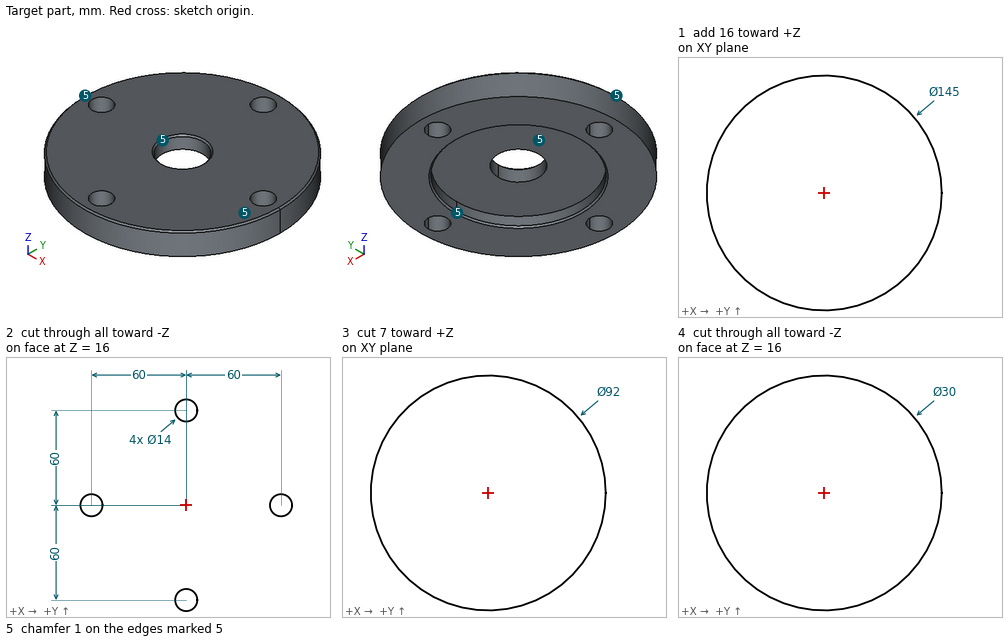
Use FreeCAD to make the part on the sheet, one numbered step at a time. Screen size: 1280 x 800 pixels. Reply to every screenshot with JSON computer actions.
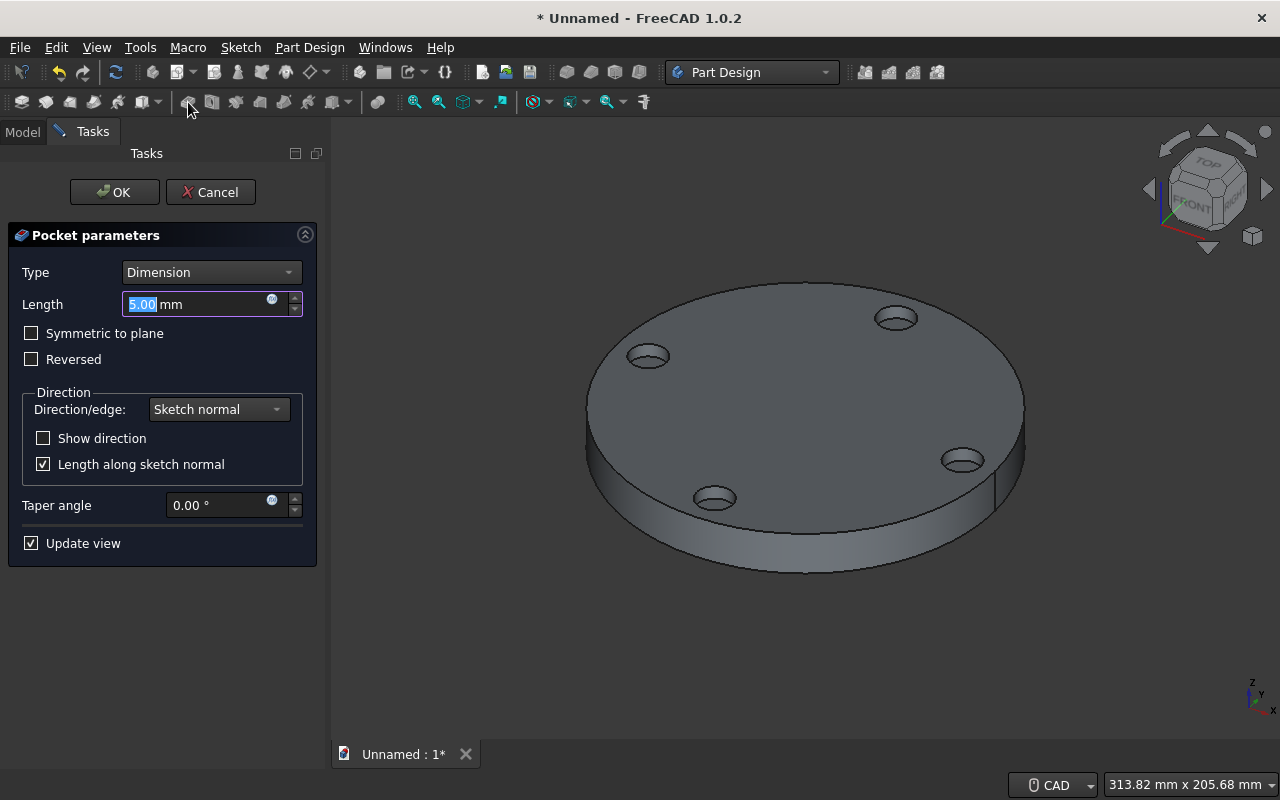
{"action": "left_click", "coordinate": [212, 272]}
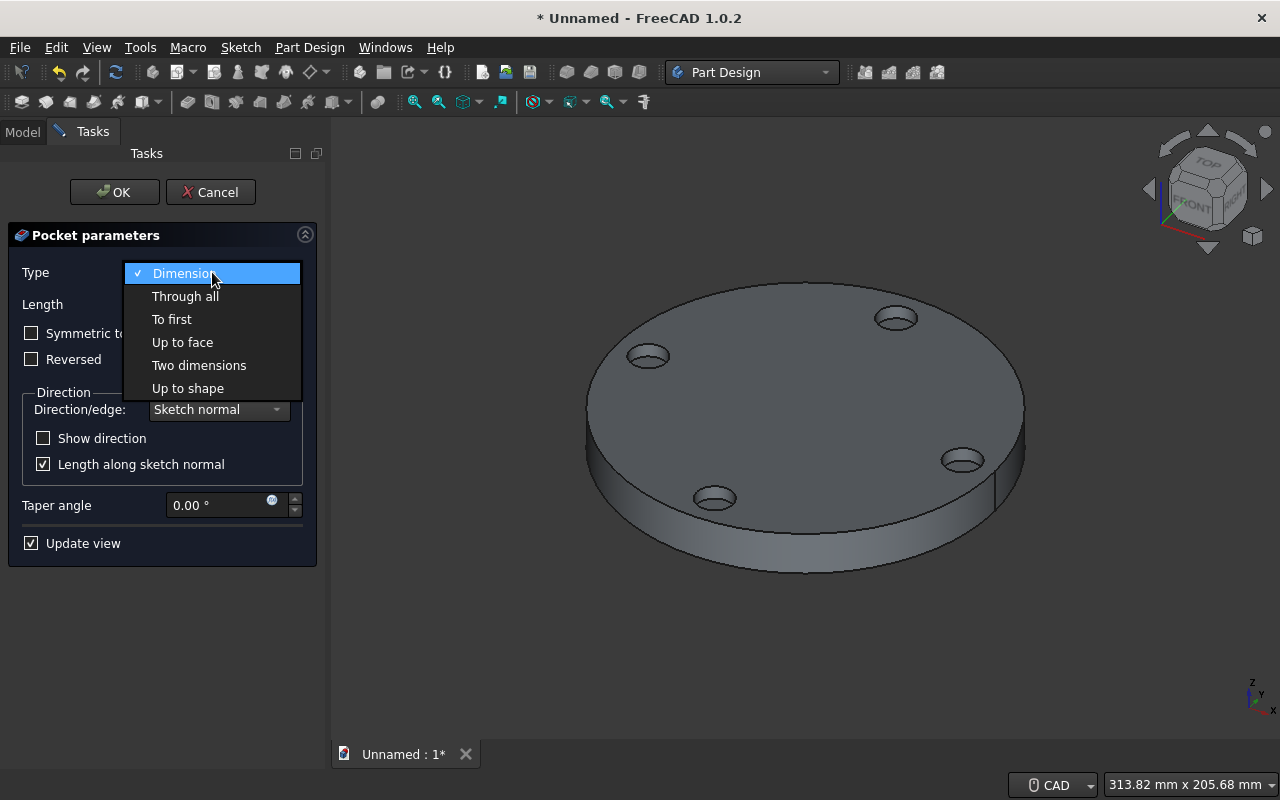
{"action": "left_click", "coordinate": [212, 296]}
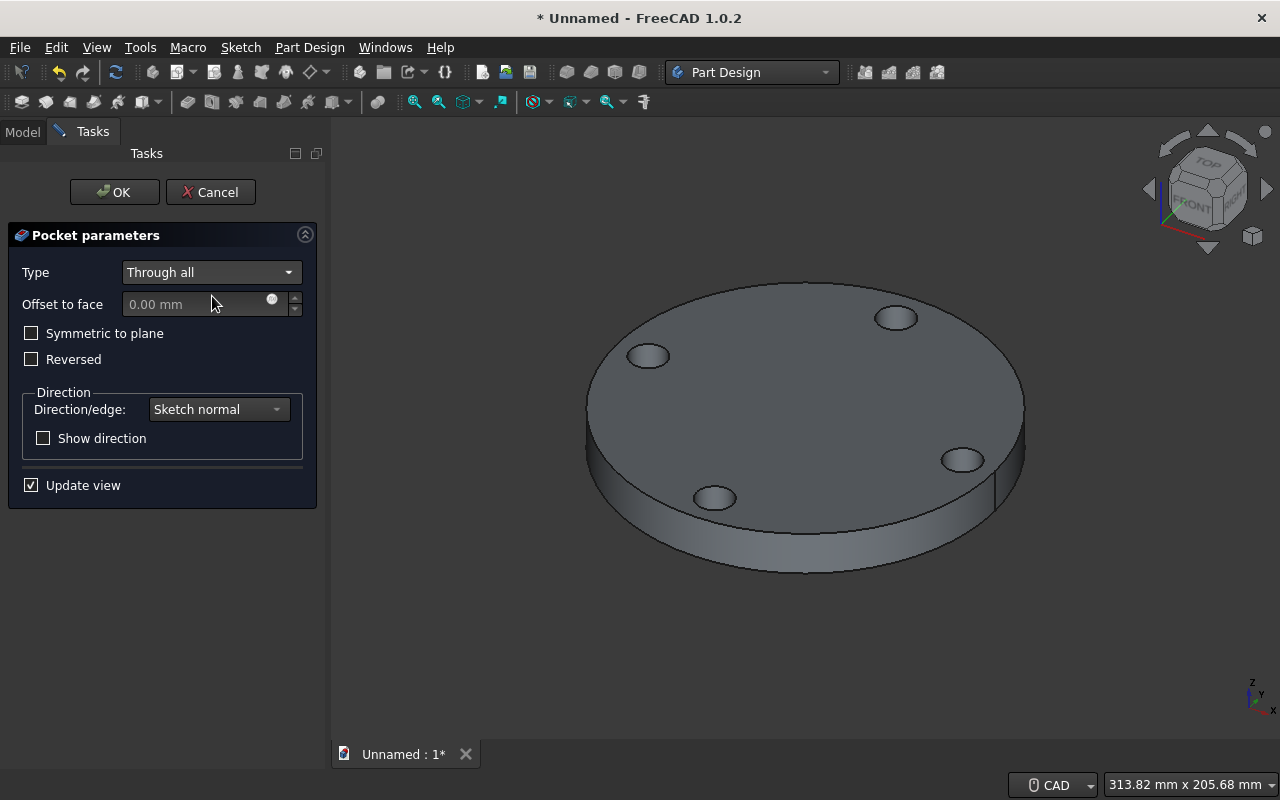
{"action": "left_click", "coordinate": [115, 192]}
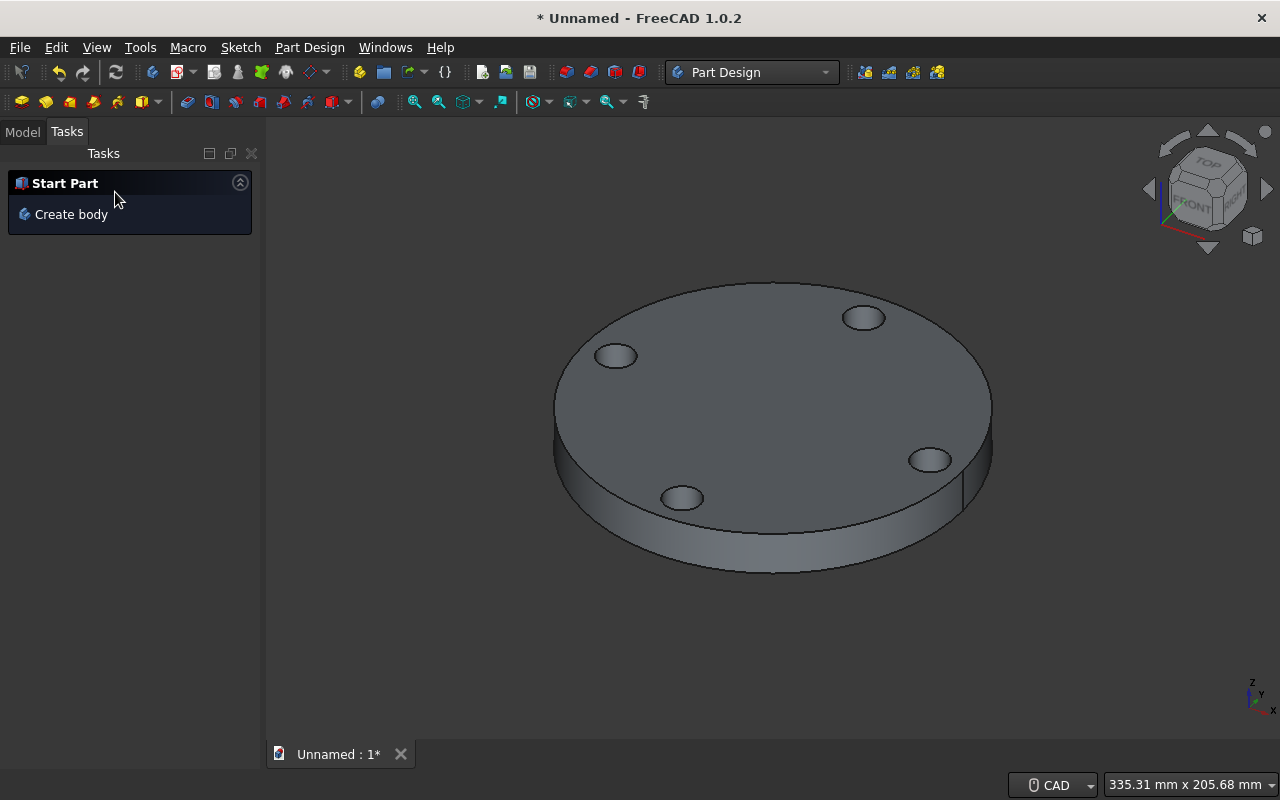
{"action": "left_click", "coordinate": [178, 72]}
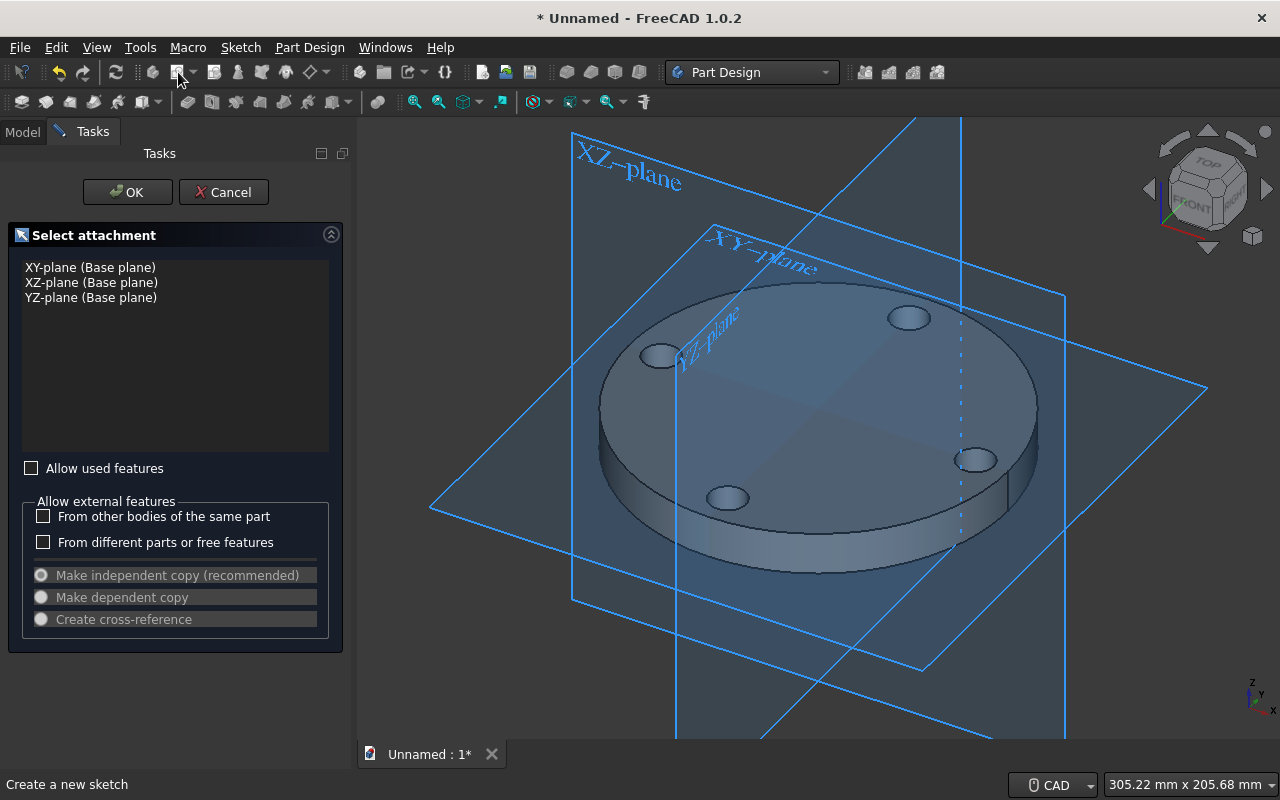
{"action": "left_click", "coordinate": [82, 268]}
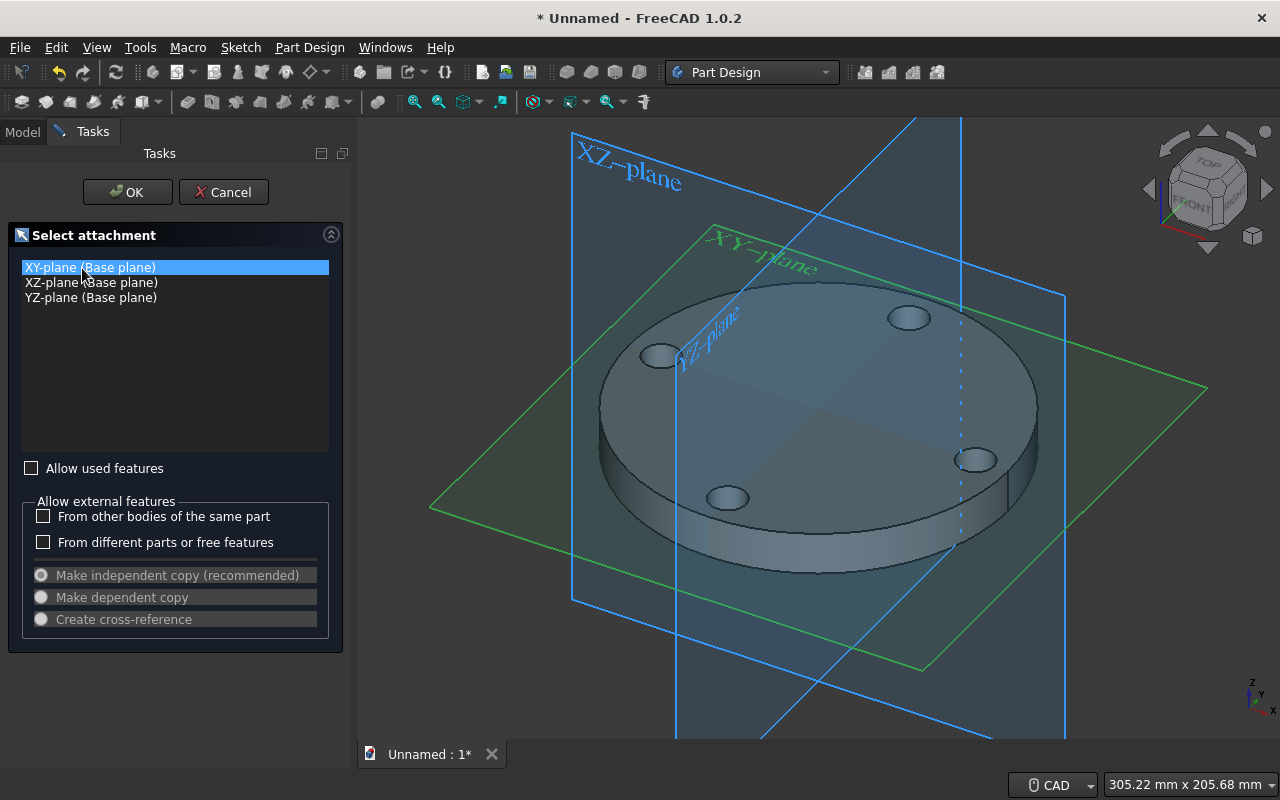
{"action": "left_click", "coordinate": [128, 192]}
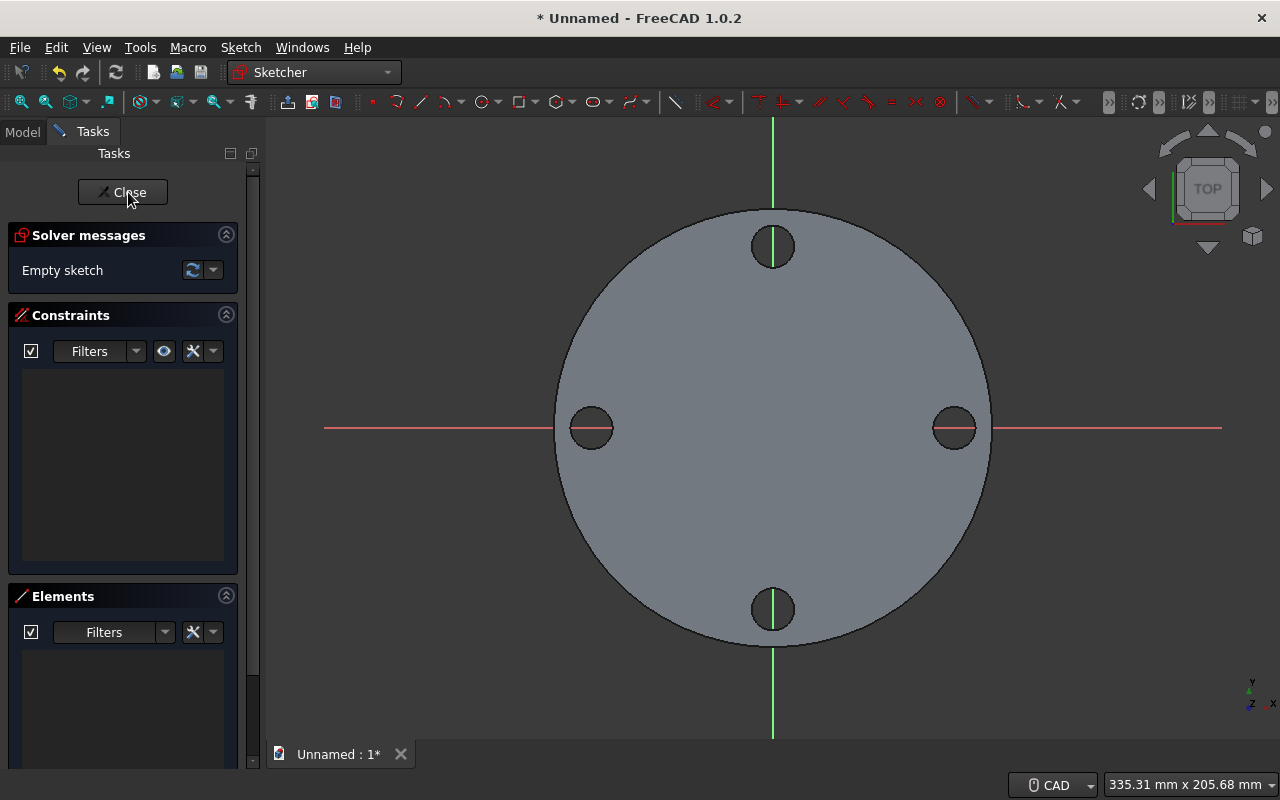
{"action": "key", "text": "q s"}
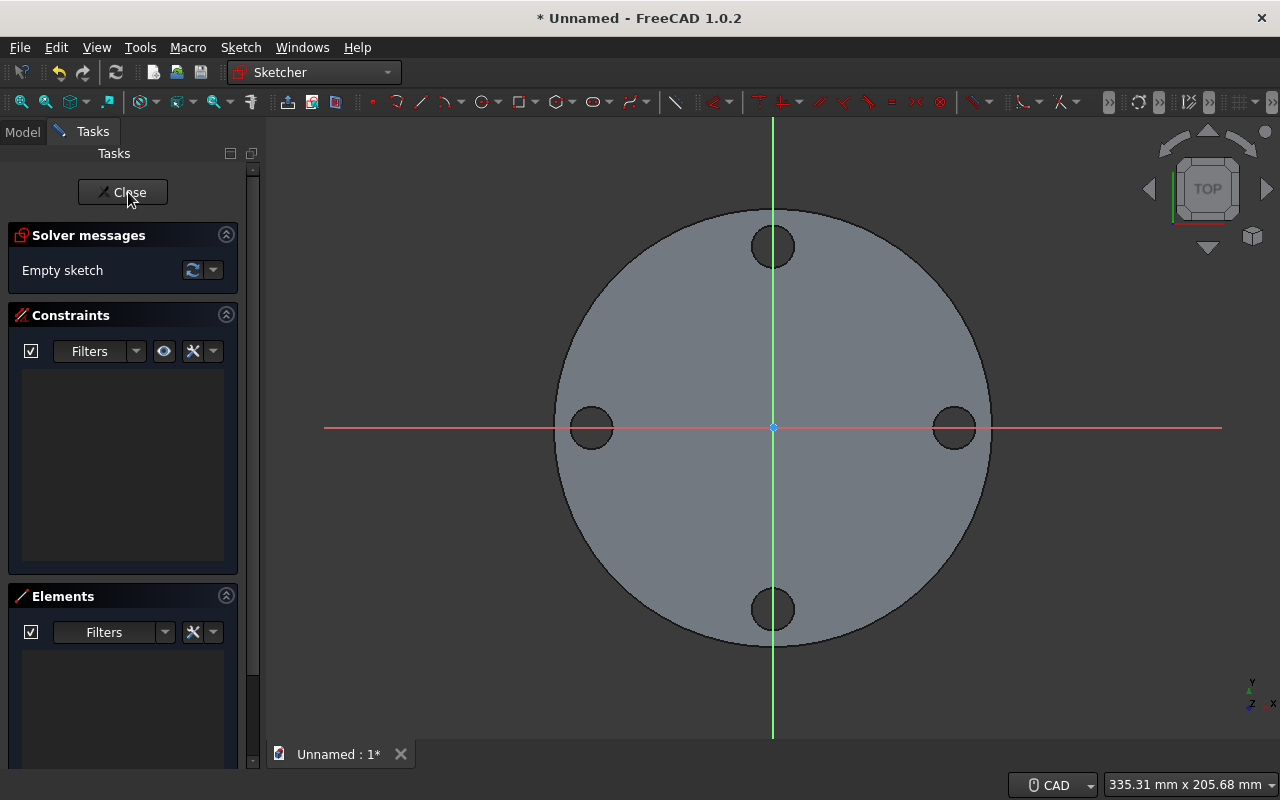
{"action": "scroll", "coordinate": [912, 428], "scroll_direction": "up", "scroll_amount": 2}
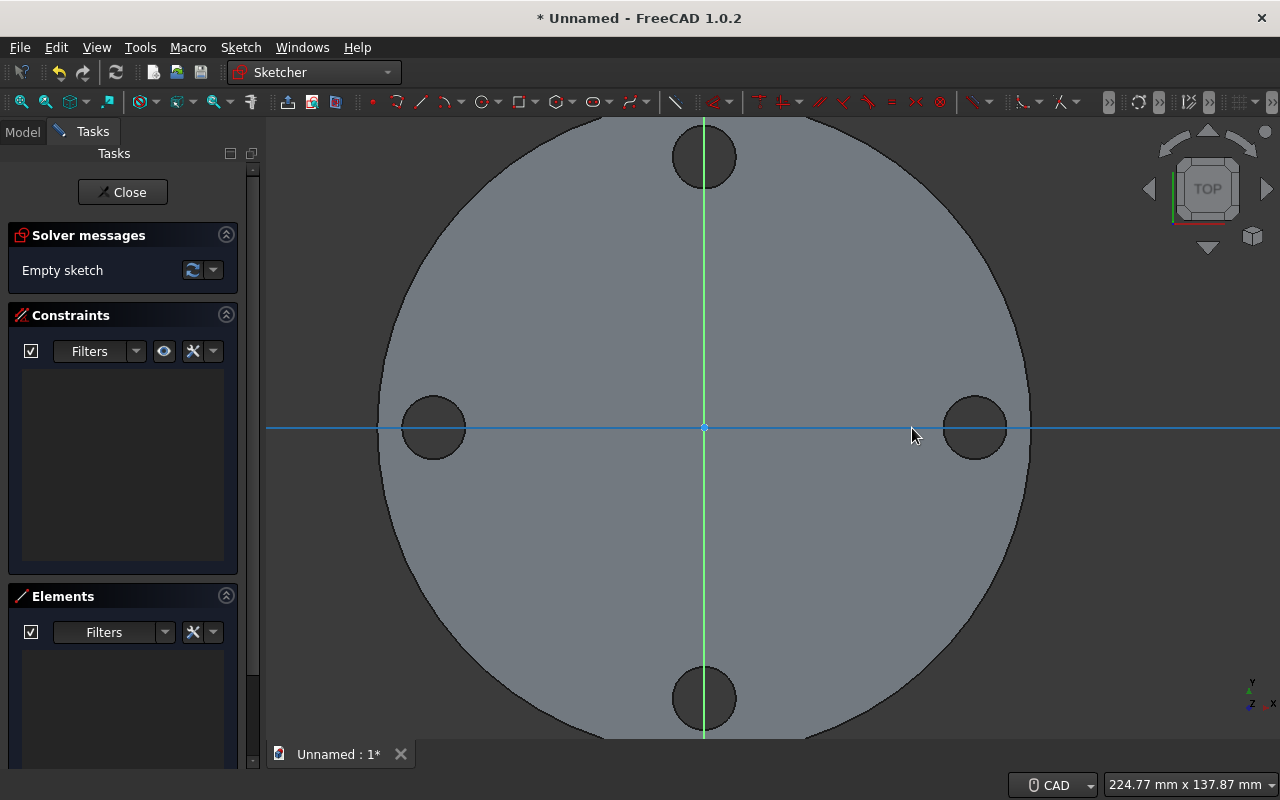
{"action": "left_click", "coordinate": [482, 102]}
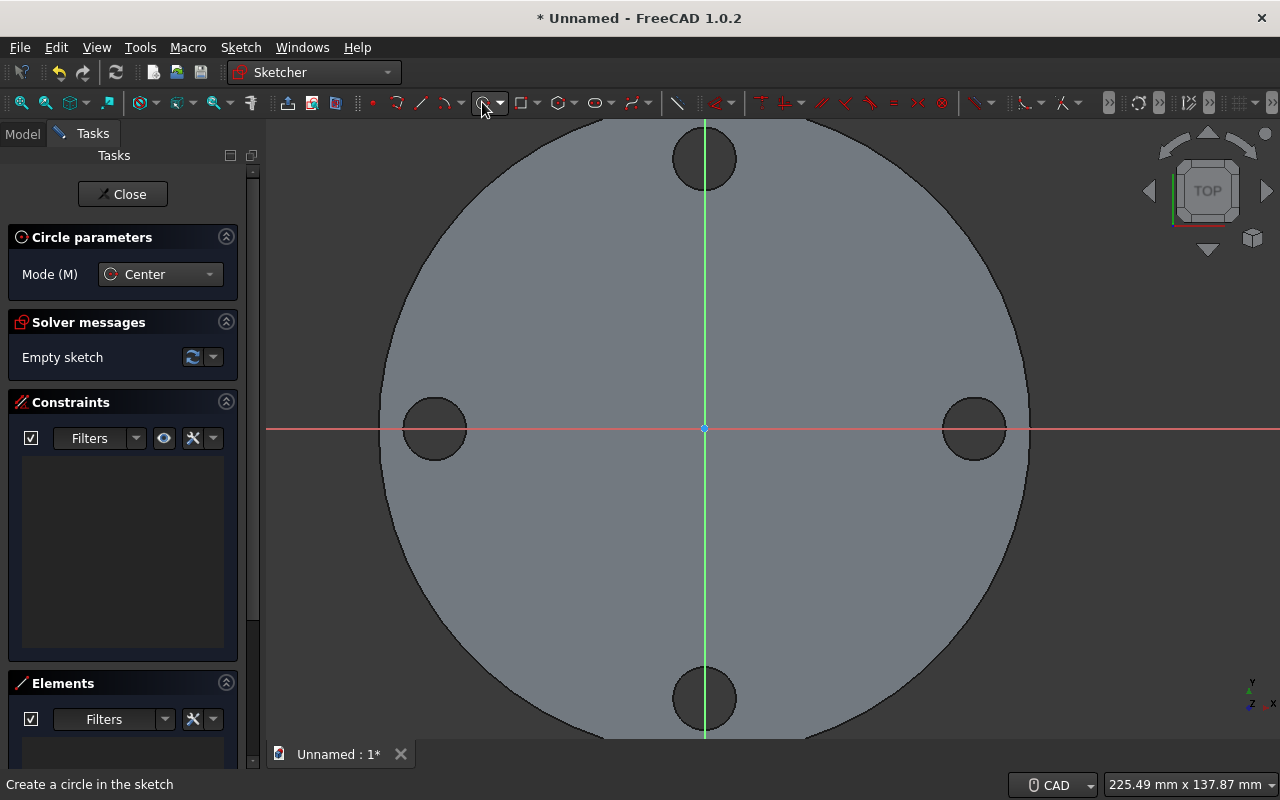
{"action": "left_click", "coordinate": [705, 429]}
{"action": "left_click", "coordinate": [851, 282]}
{"action": "key", "text": "Escape"}